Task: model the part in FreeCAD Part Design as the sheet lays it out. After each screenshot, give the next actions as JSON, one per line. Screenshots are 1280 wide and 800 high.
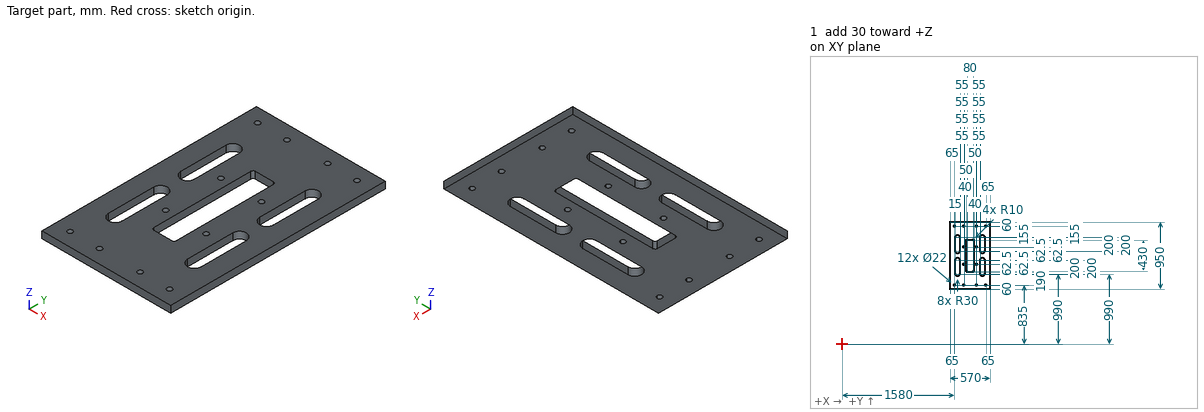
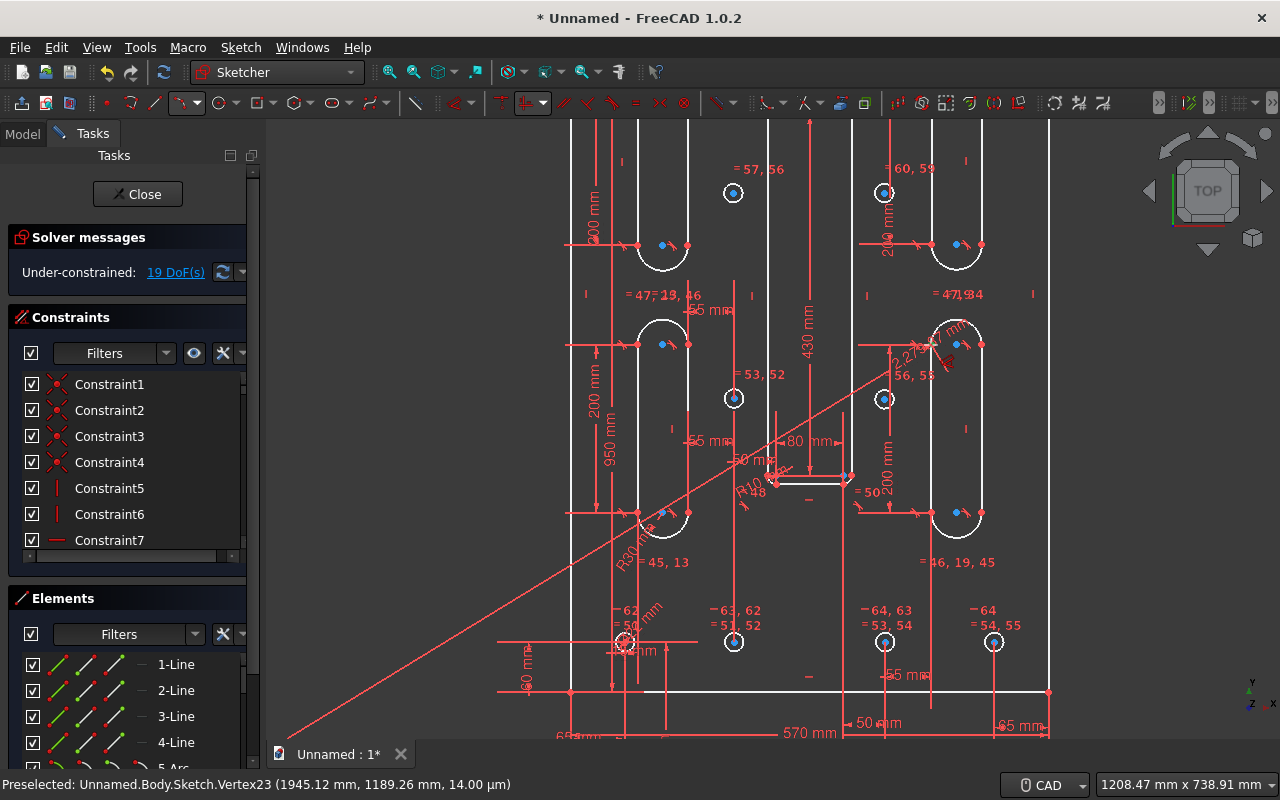
{"action": "left_click", "coordinate": [885, 399]}
{"action": "left_click", "coordinate": [908, 311]}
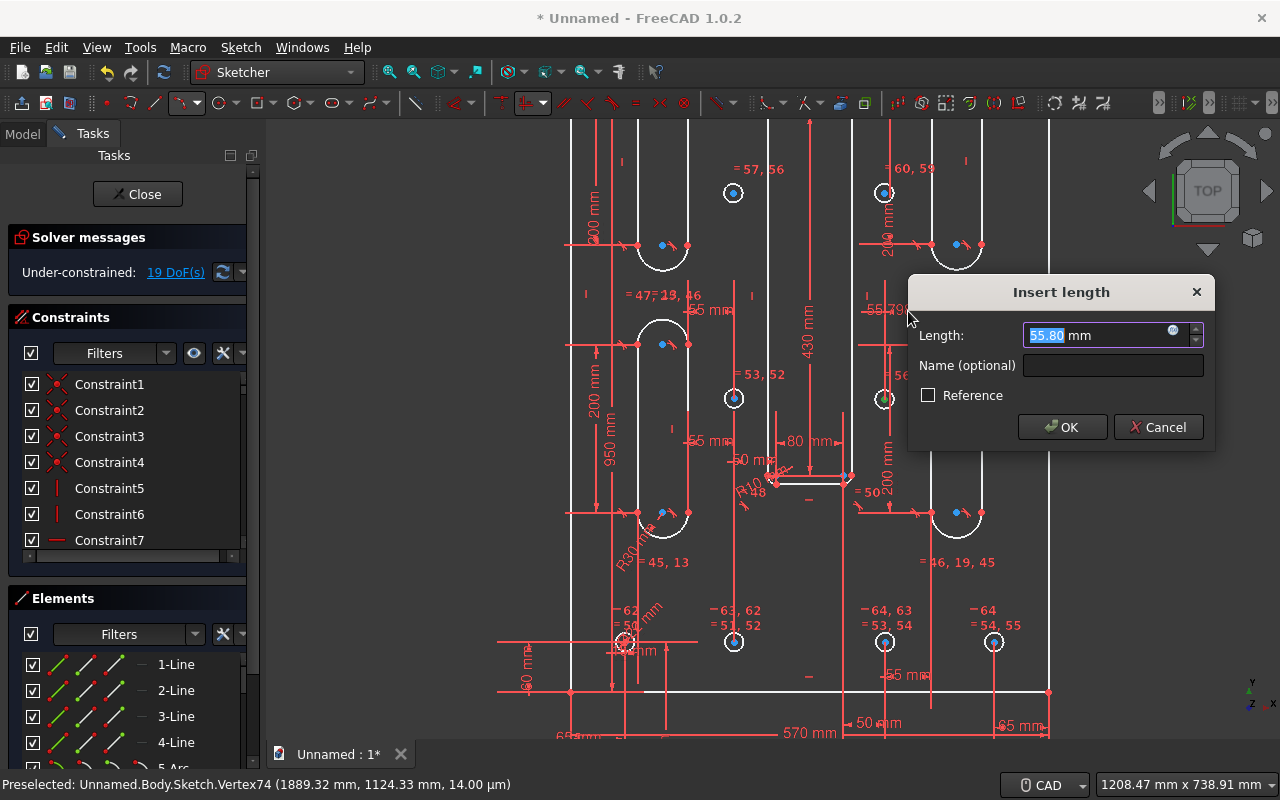
{"action": "type", "text": "55"}
{"action": "key", "text": "Return"}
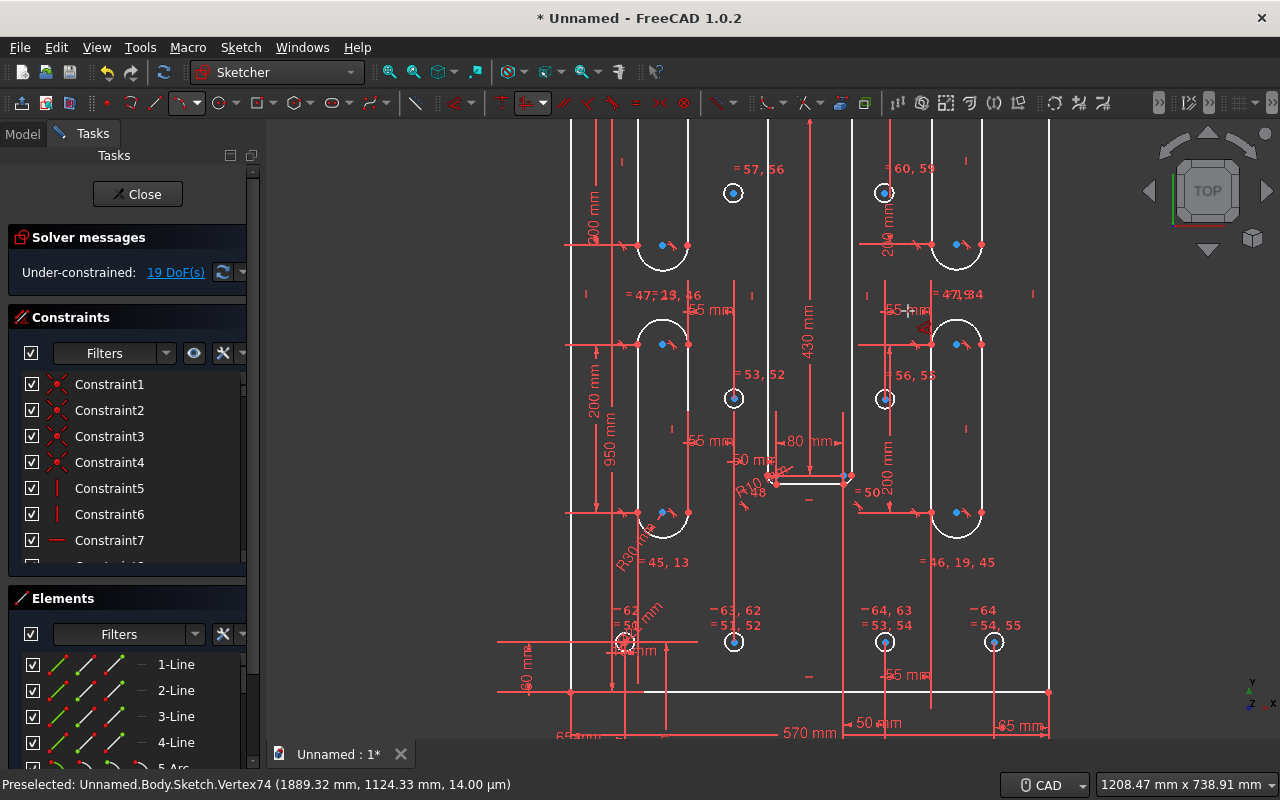
{"action": "left_click", "coordinate": [688, 245]}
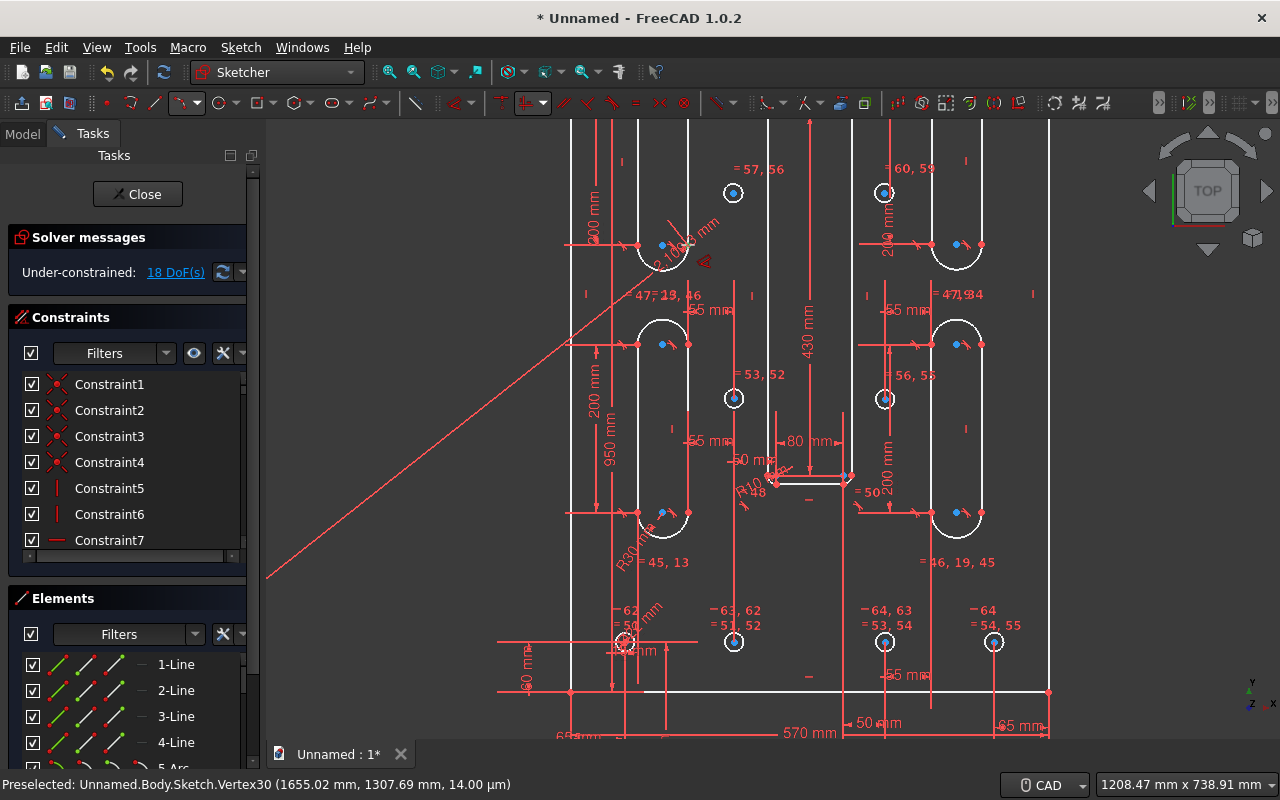
{"action": "left_click", "coordinate": [733, 193]}
{"action": "left_click", "coordinate": [711, 159]}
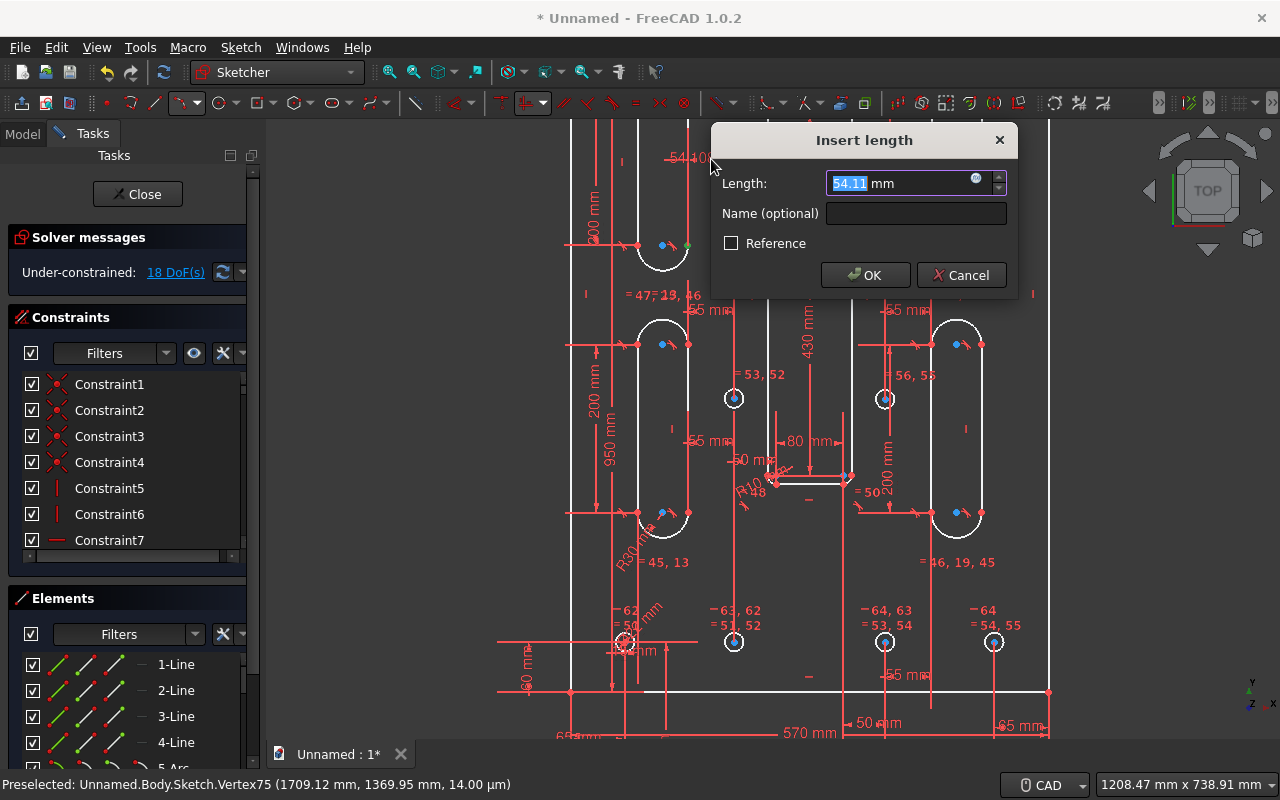
{"action": "type", "text": "55"}
{"action": "key", "text": "Return"}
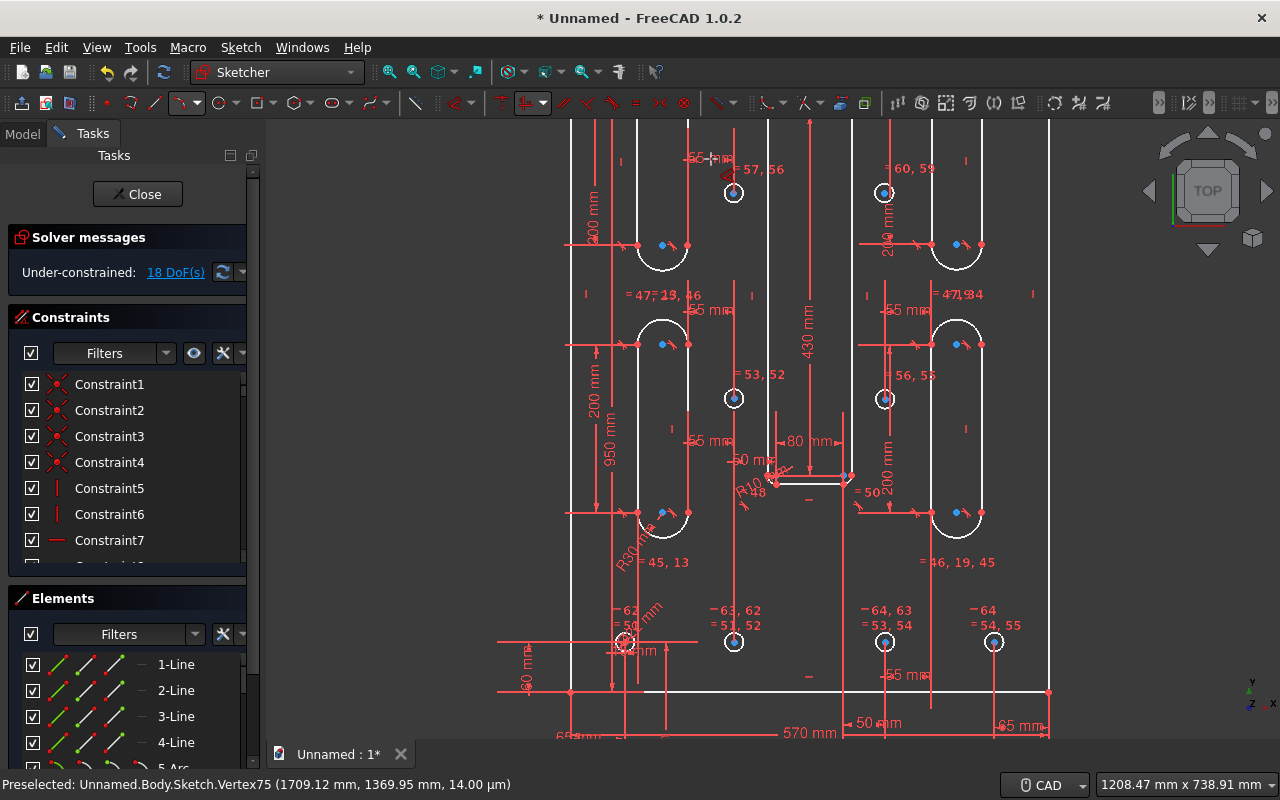
{"action": "scroll", "coordinate": [933, 347], "scroll_direction": "down", "scroll_amount": 6}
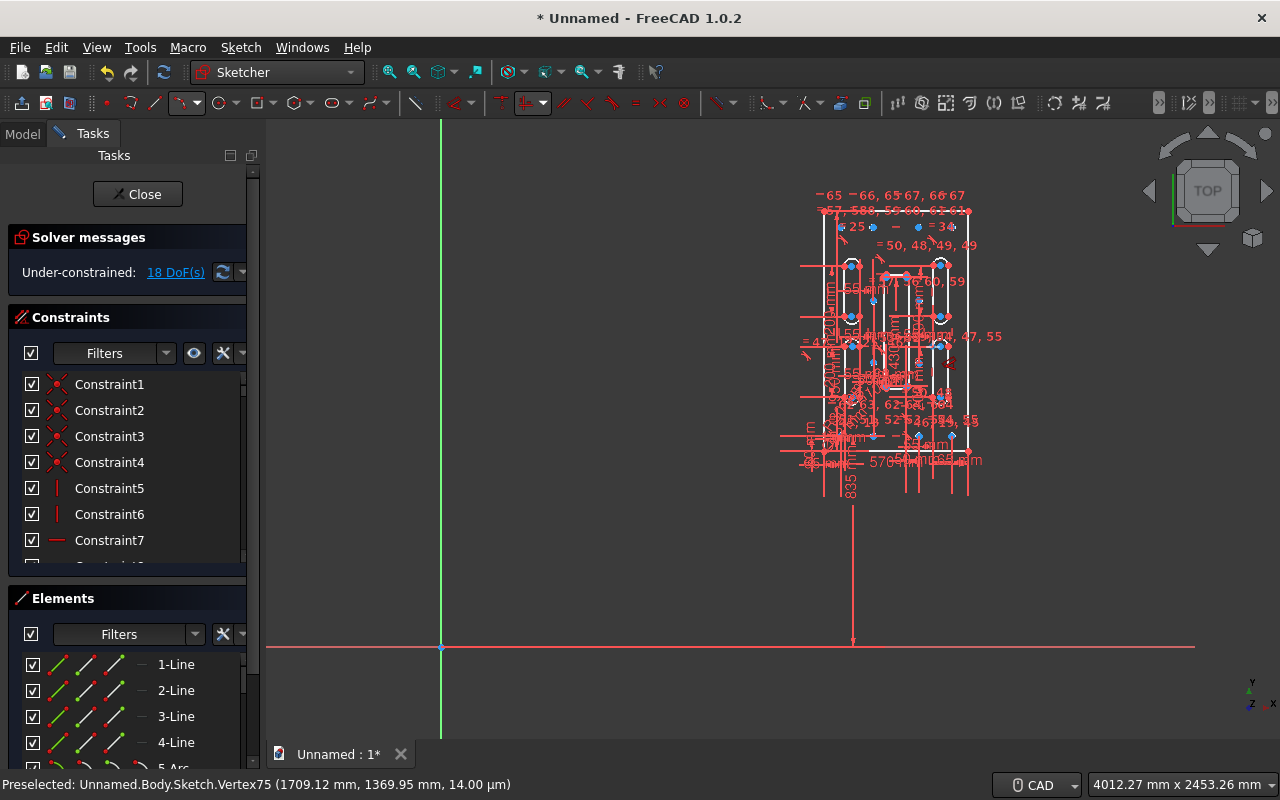
{"action": "scroll", "coordinate": [884, 277], "scroll_direction": "up", "scroll_amount": 8}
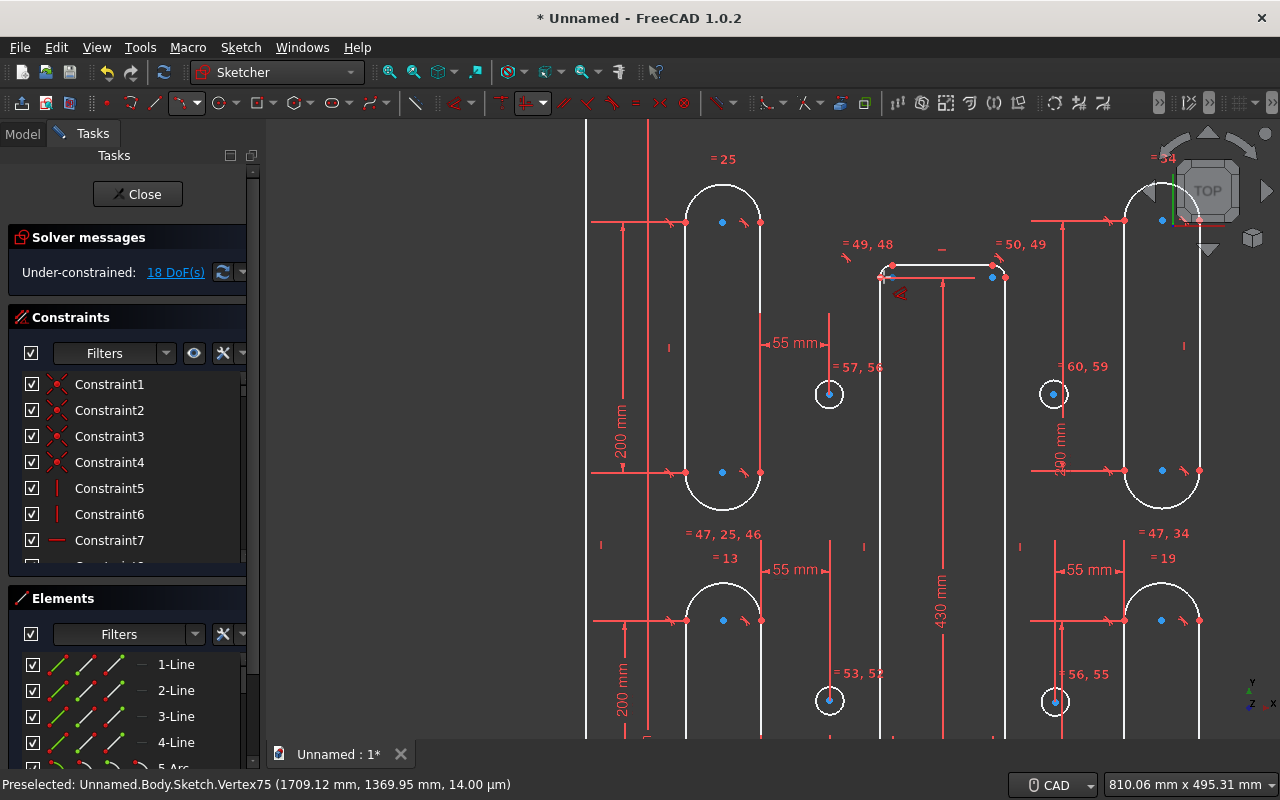
{"action": "left_click", "coordinate": [880, 278]}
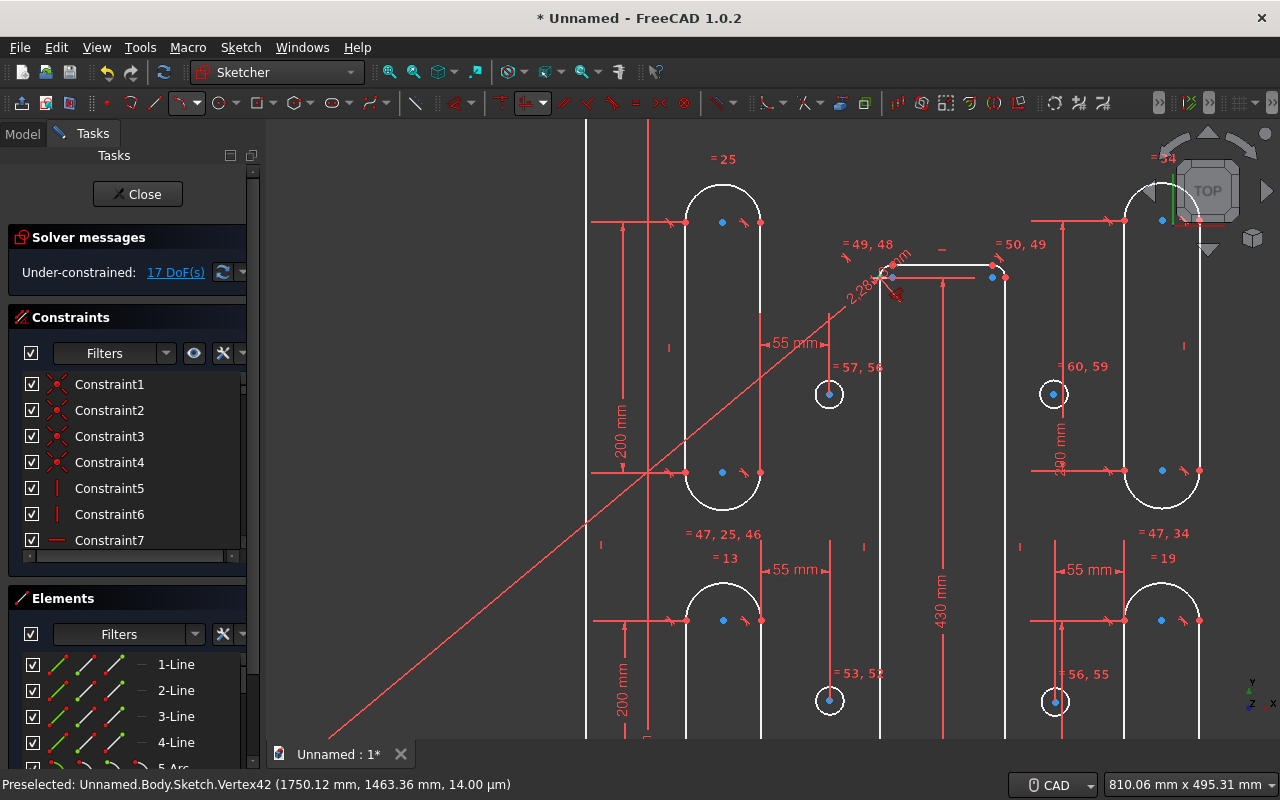
{"action": "left_click", "coordinate": [829, 395]}
{"action": "left_click", "coordinate": [855, 244]}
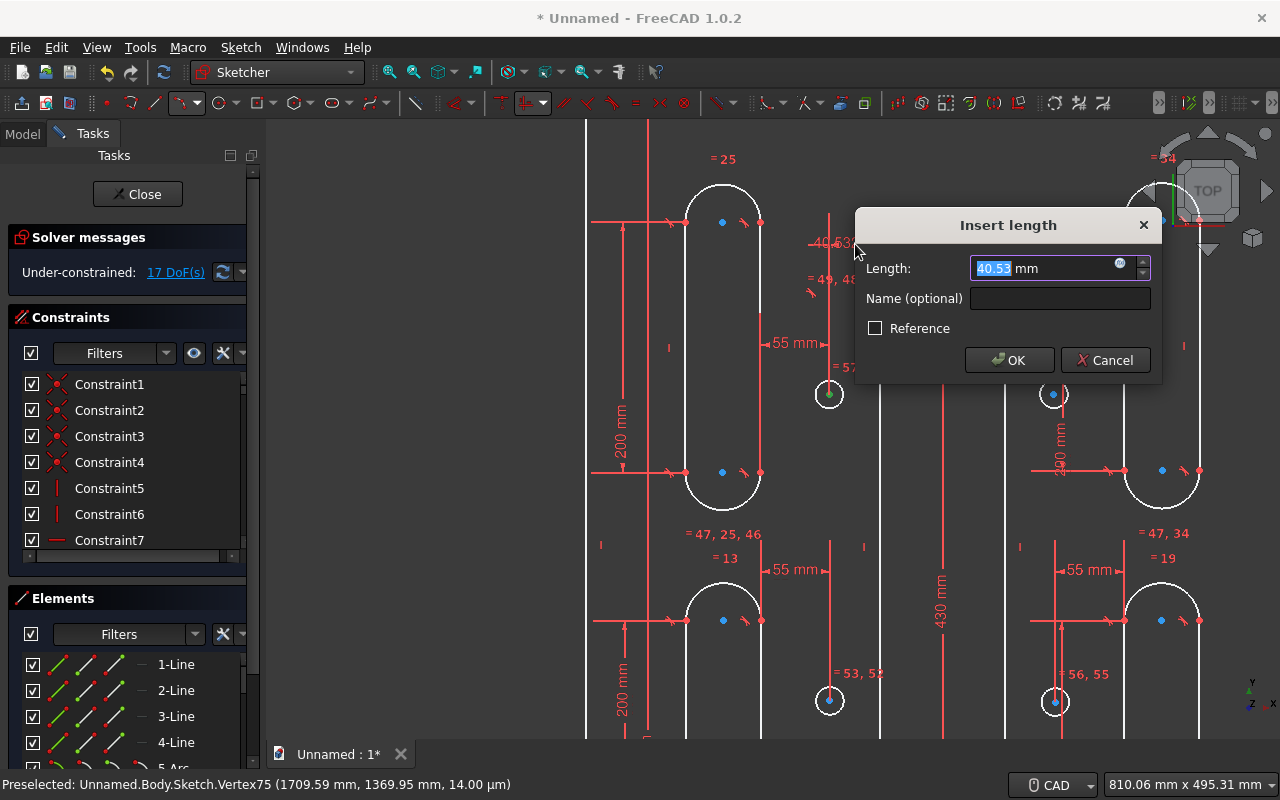
{"action": "type", "text": "40"}
{"action": "key", "text": "Return"}